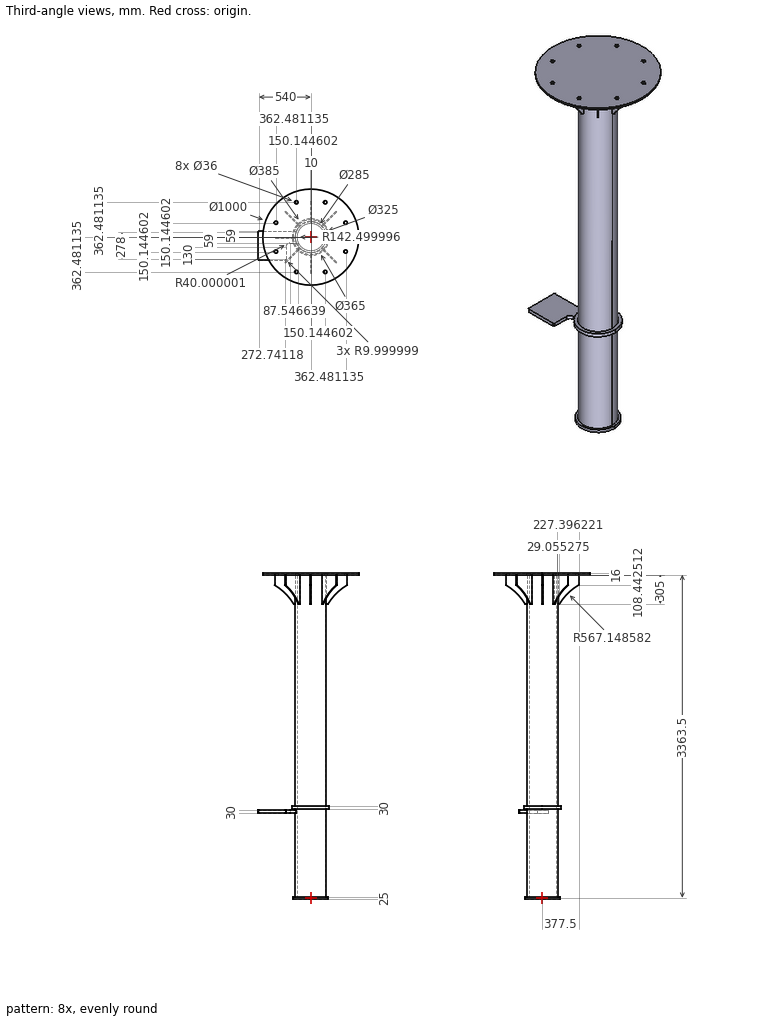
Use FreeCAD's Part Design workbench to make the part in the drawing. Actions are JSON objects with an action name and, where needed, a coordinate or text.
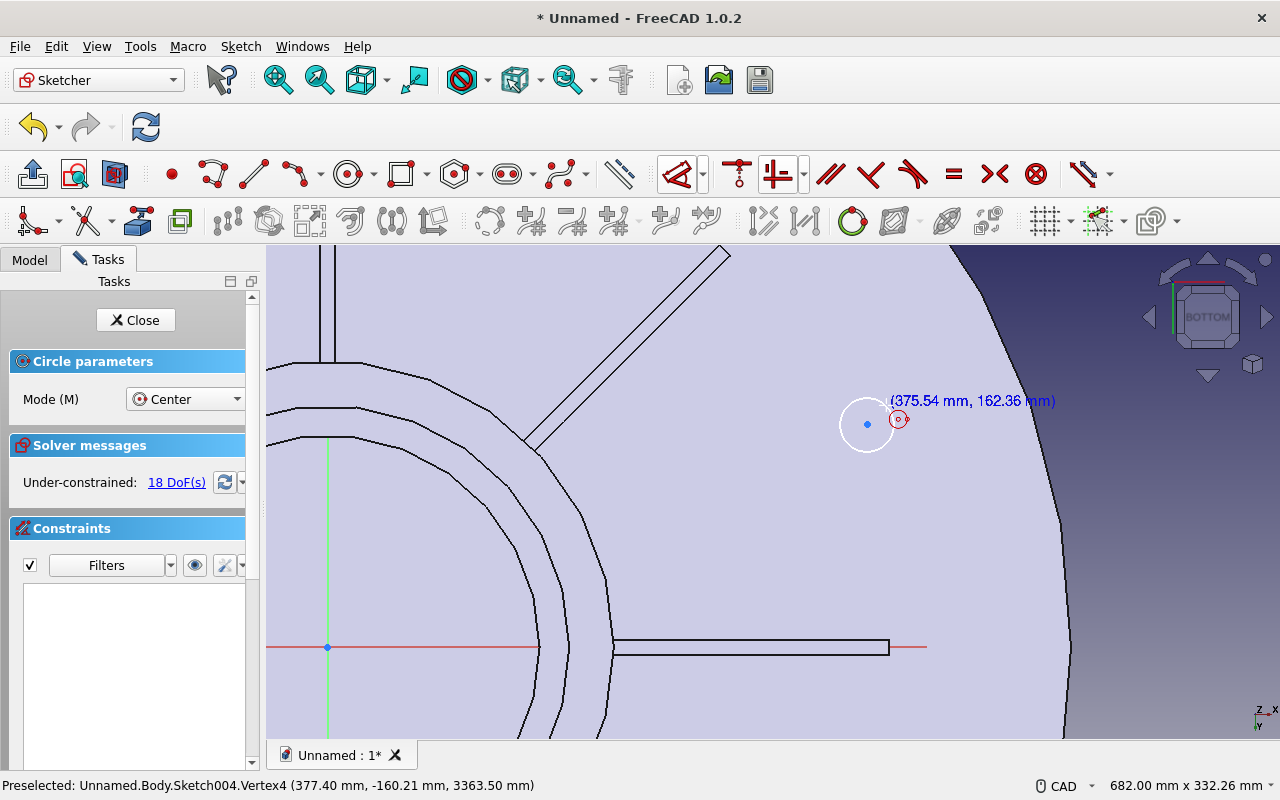
{"action": "scroll", "coordinate": [867, 425], "scroll_direction": "down", "scroll_amount": 6}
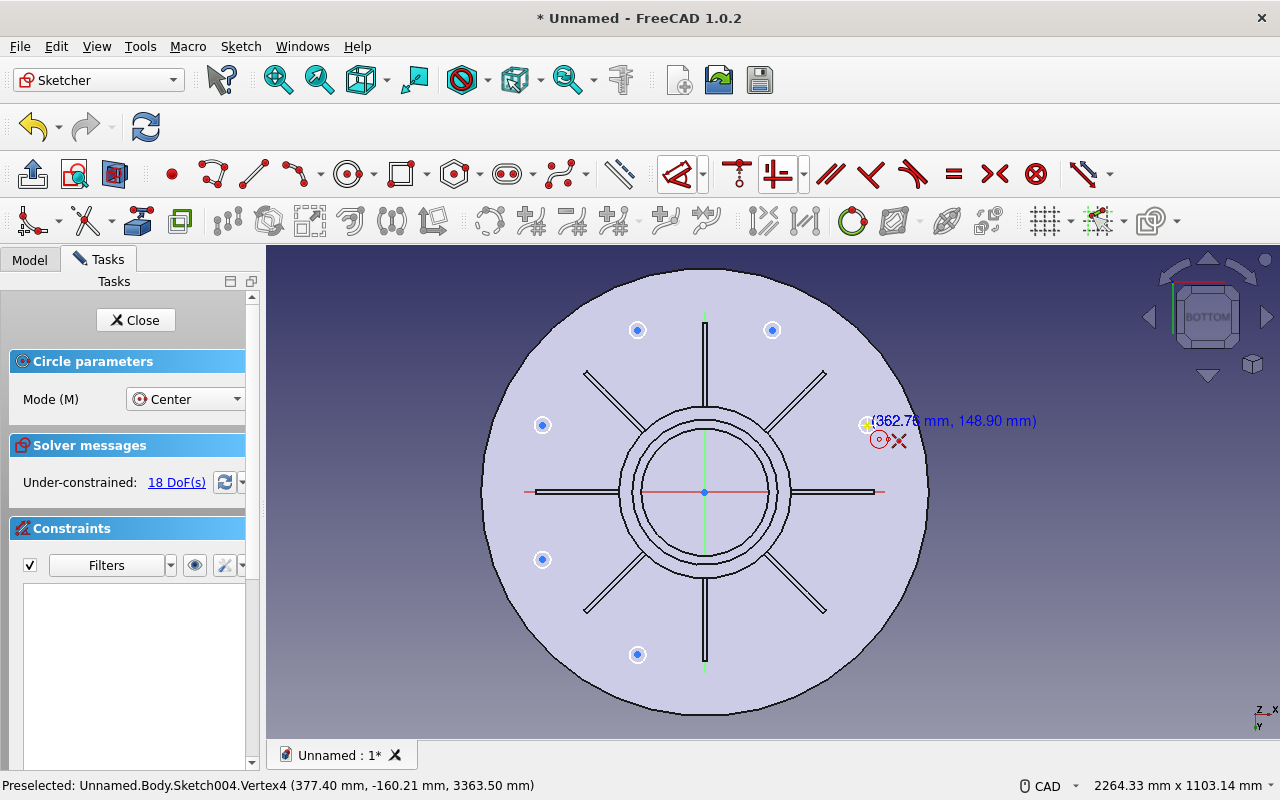
{"action": "scroll", "coordinate": [867, 559], "scroll_direction": "up", "scroll_amount": 6}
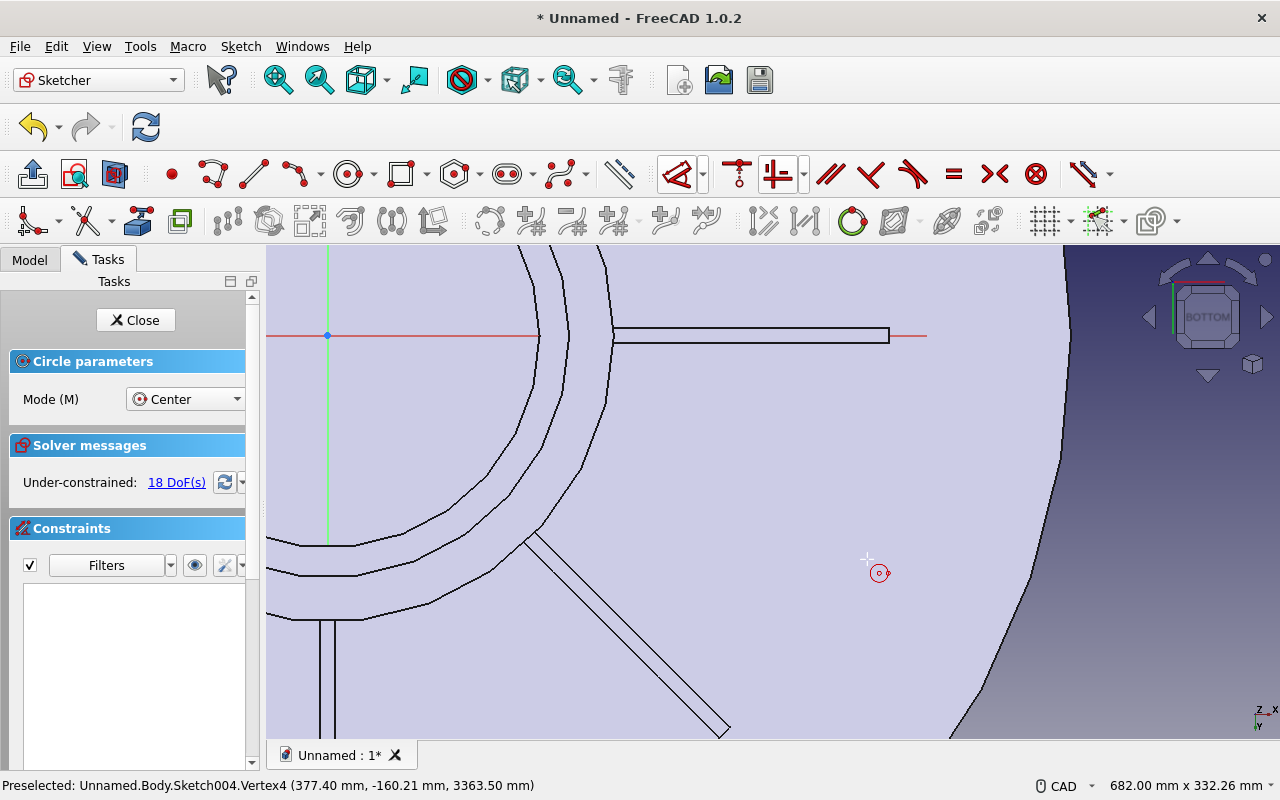
{"action": "left_click", "coordinate": [867, 559]}
{"action": "left_click", "coordinate": [886, 540]}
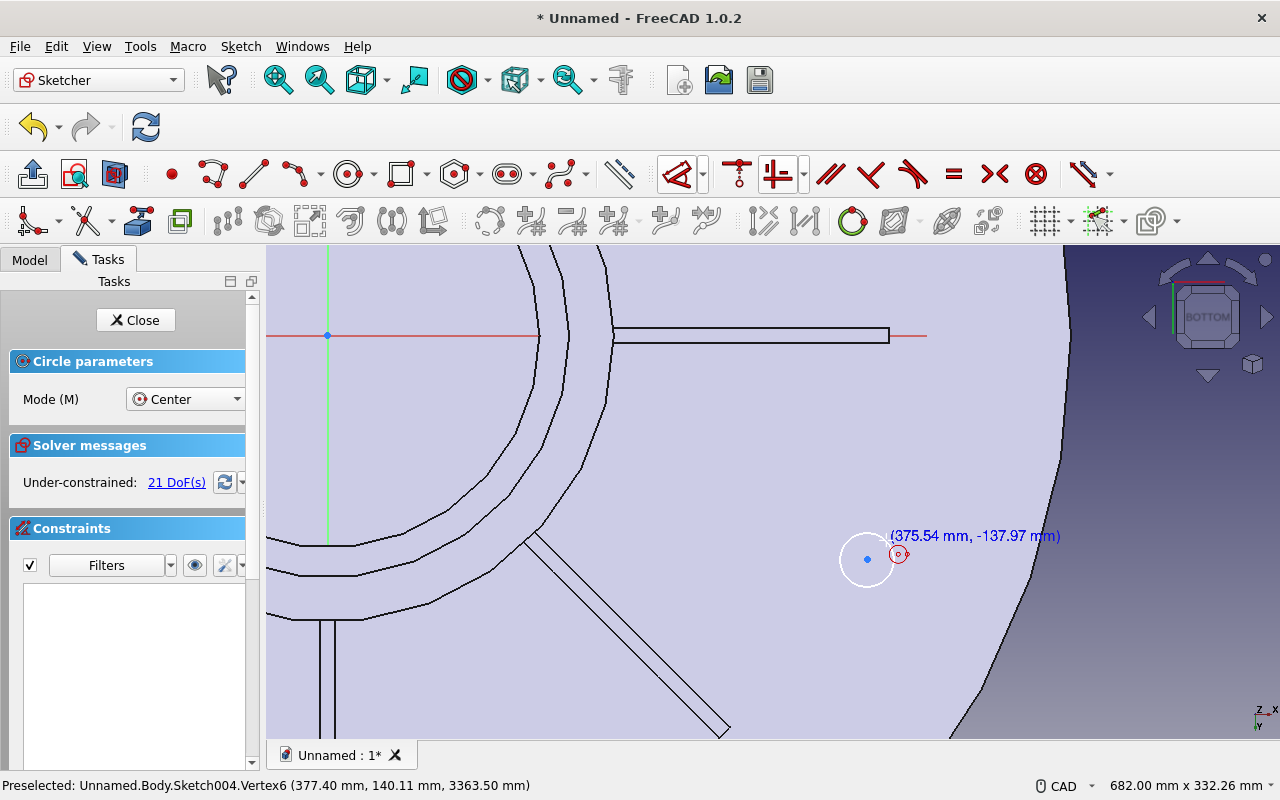
{"action": "scroll", "coordinate": [867, 559], "scroll_direction": "down", "scroll_amount": 6}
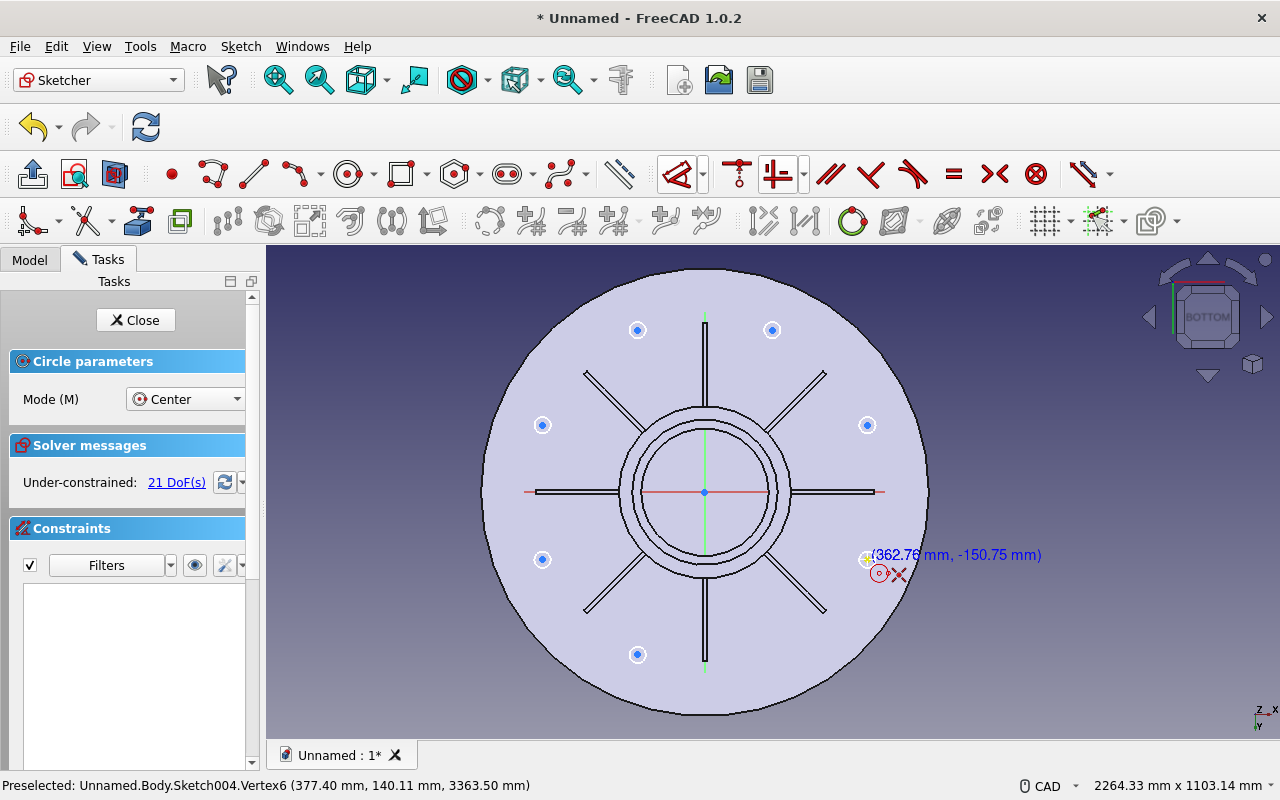
{"action": "scroll", "coordinate": [772, 655], "scroll_direction": "up", "scroll_amount": 6}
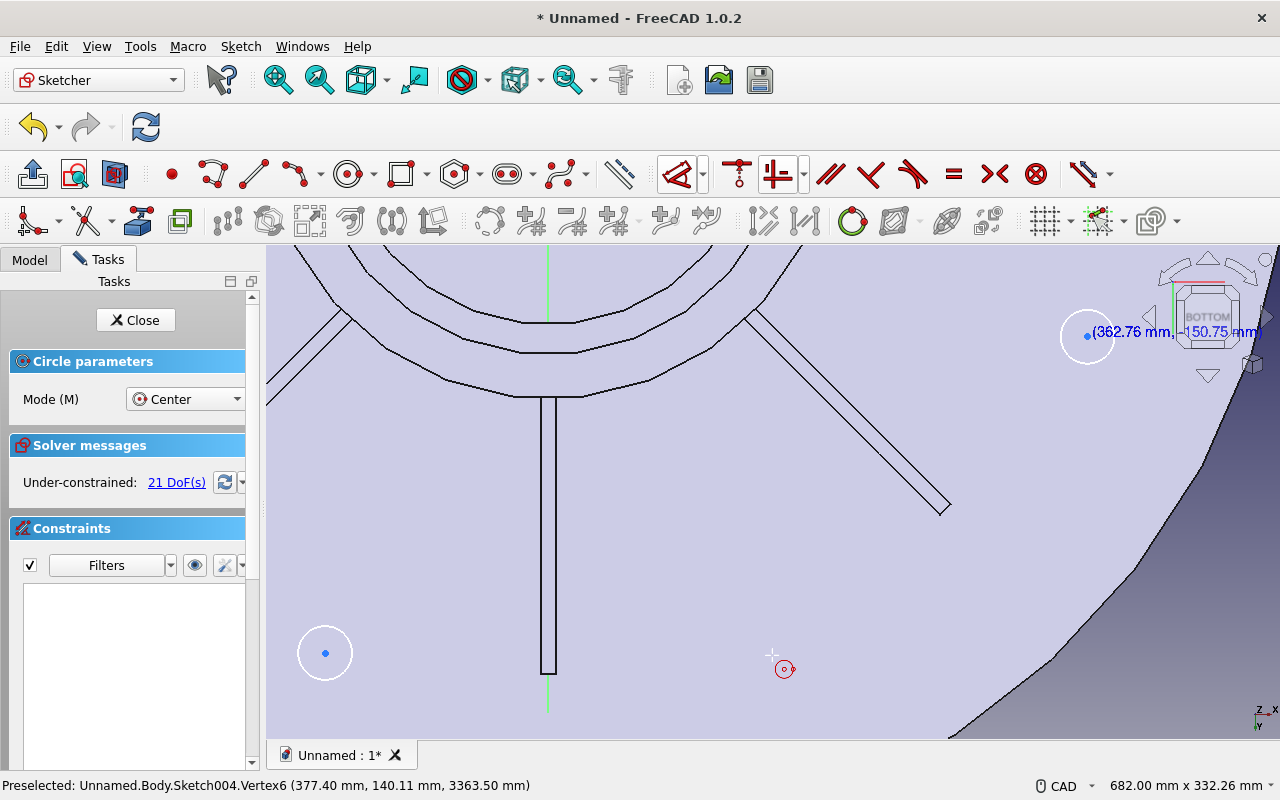
{"action": "left_click", "coordinate": [772, 652]}
{"action": "left_click", "coordinate": [790, 633]}
{"action": "key", "text": "Escape"}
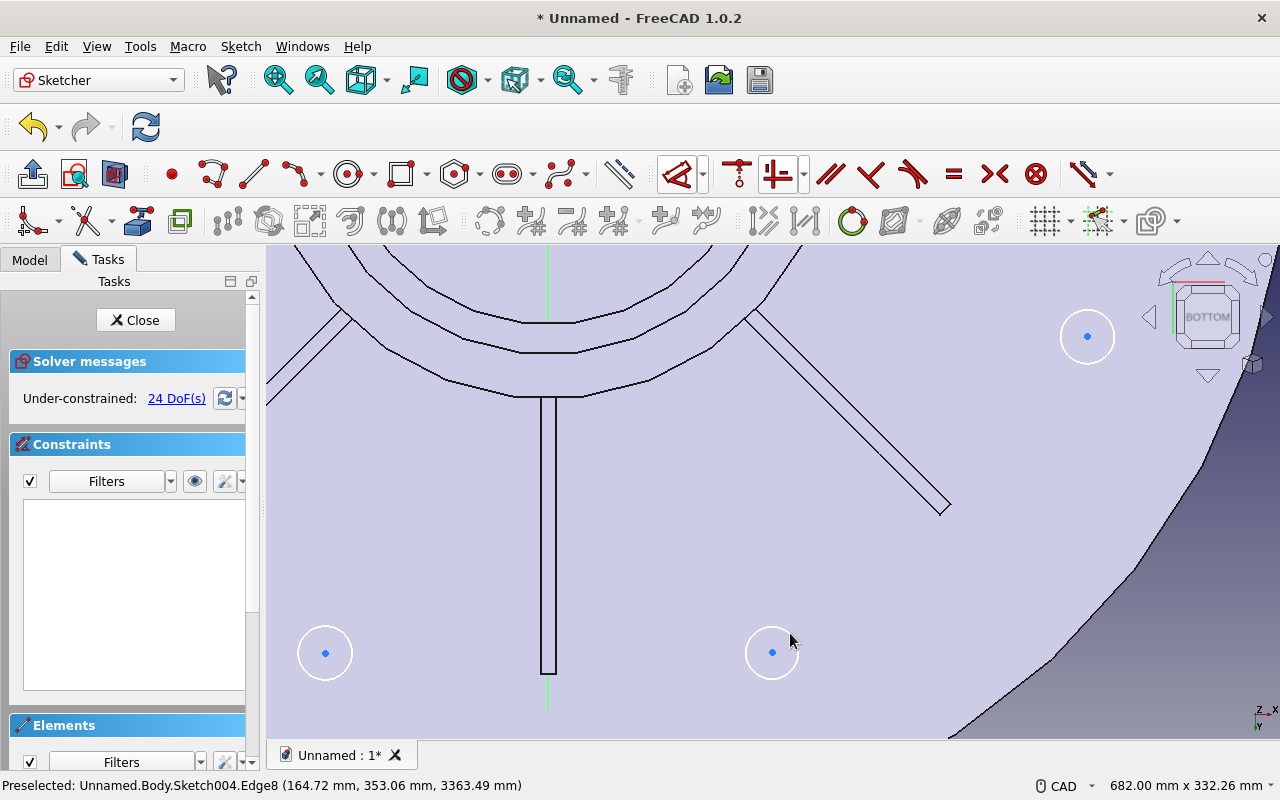
{"action": "left_click", "coordinate": [344, 634]}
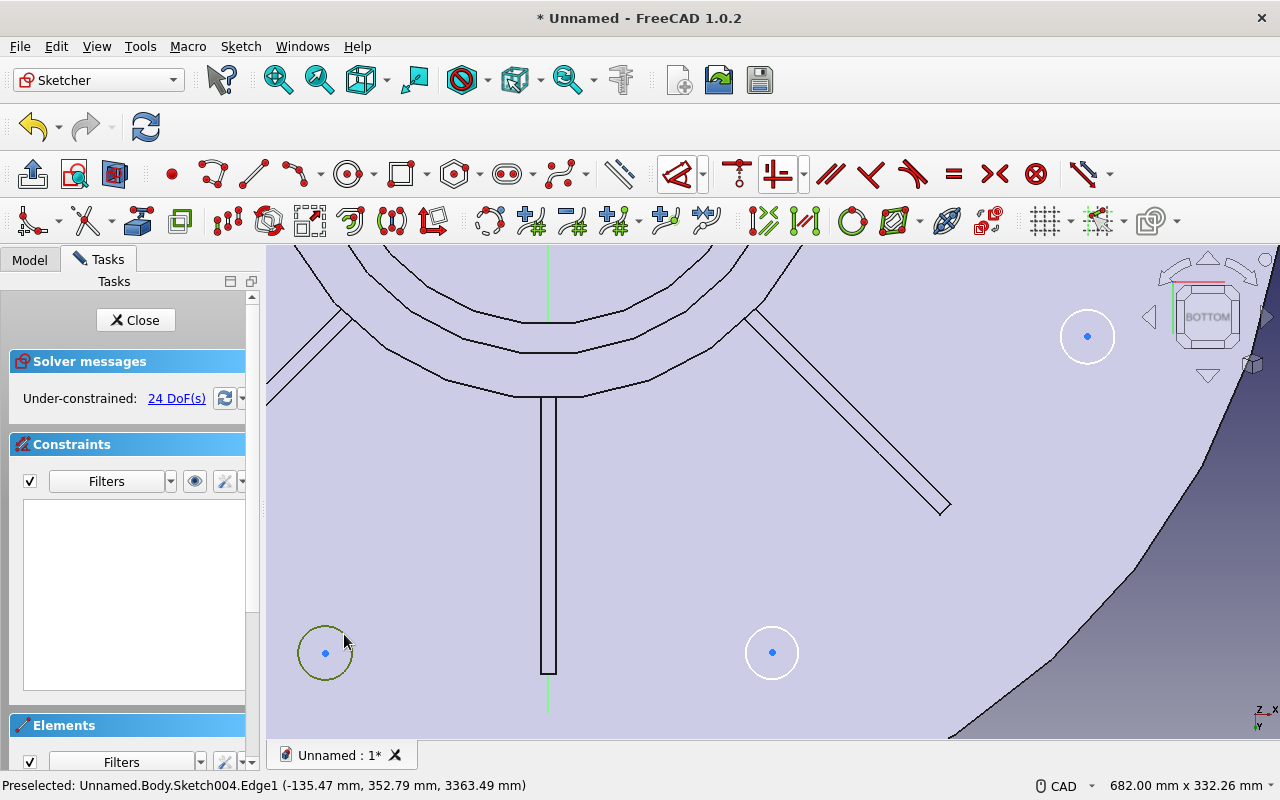
{"action": "scroll", "coordinate": [772, 655], "scroll_direction": "down", "scroll_amount": 6}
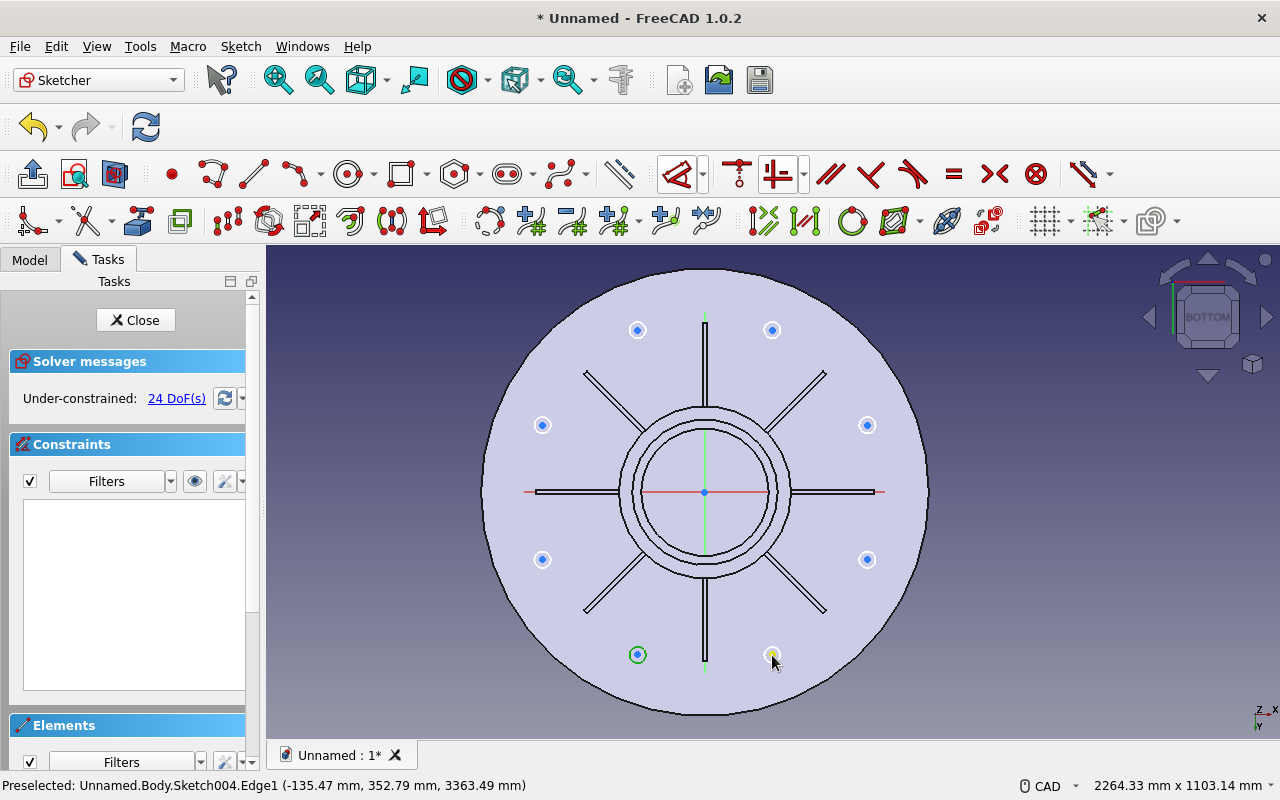
{"action": "scroll", "coordinate": [548, 554], "scroll_direction": "up", "scroll_amount": 3}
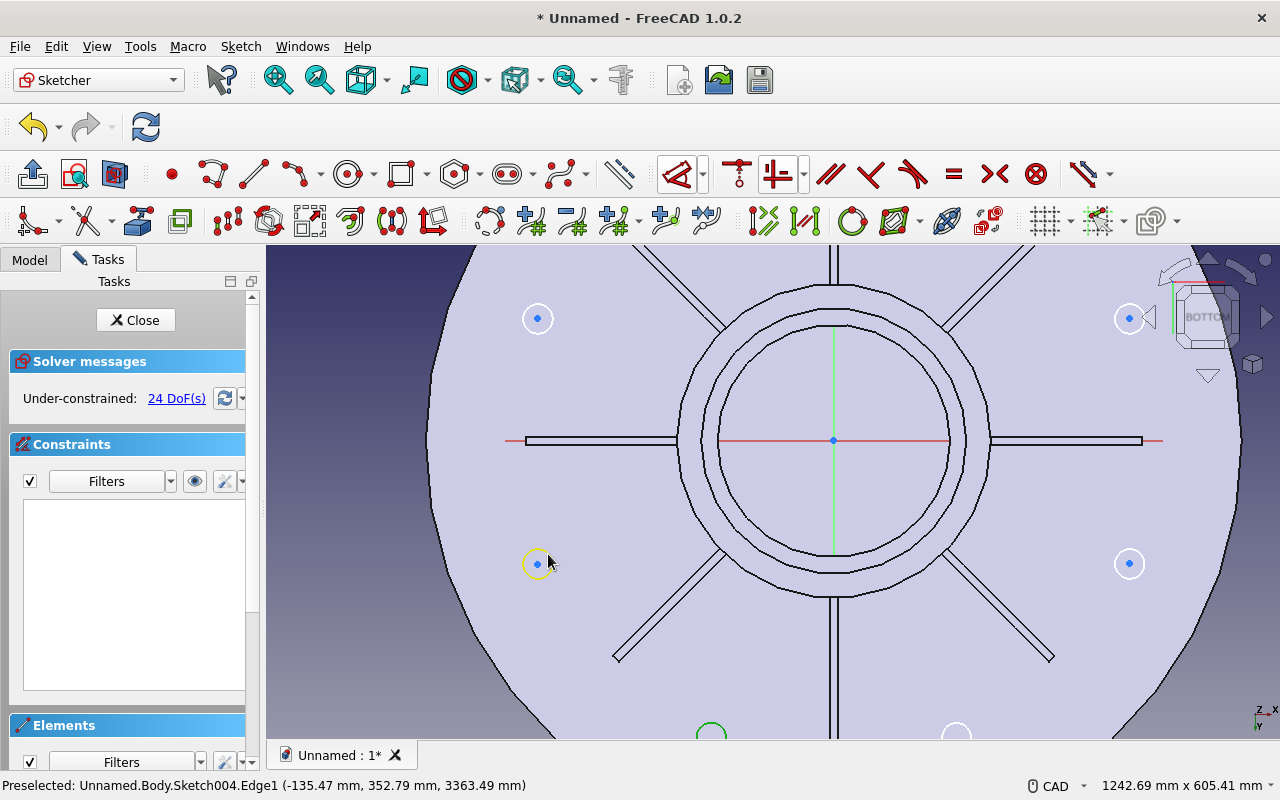
{"action": "left_click", "coordinate": [548, 554]}